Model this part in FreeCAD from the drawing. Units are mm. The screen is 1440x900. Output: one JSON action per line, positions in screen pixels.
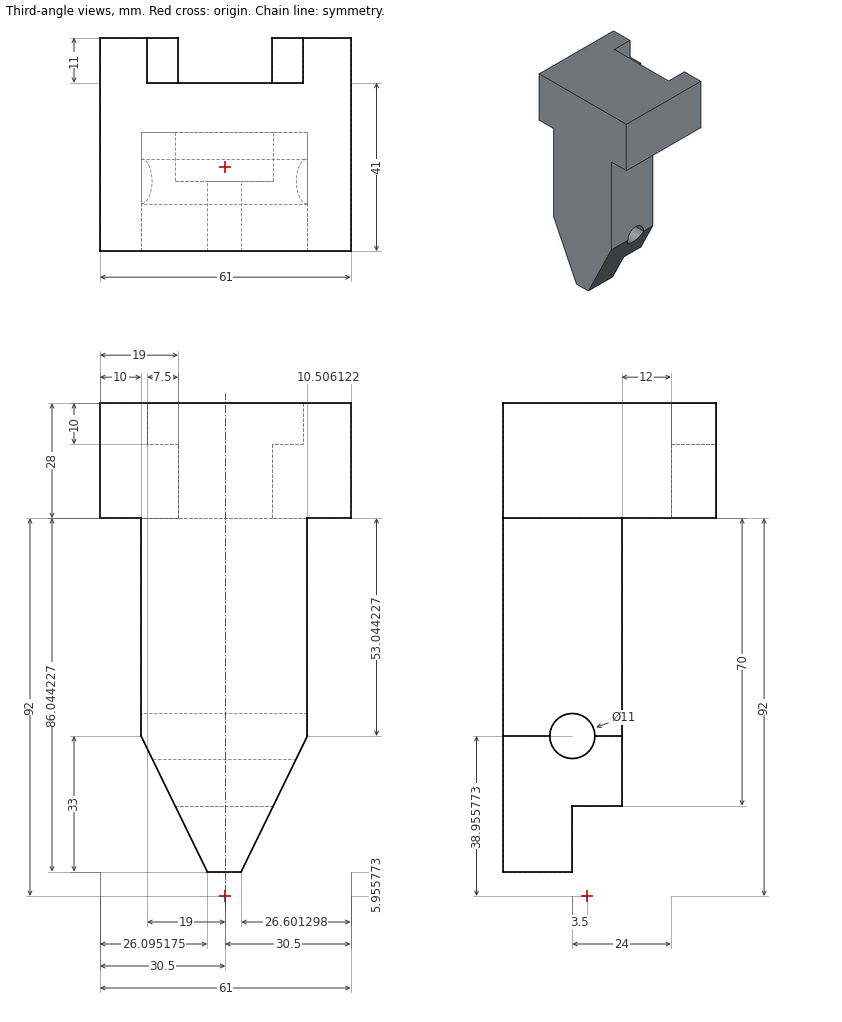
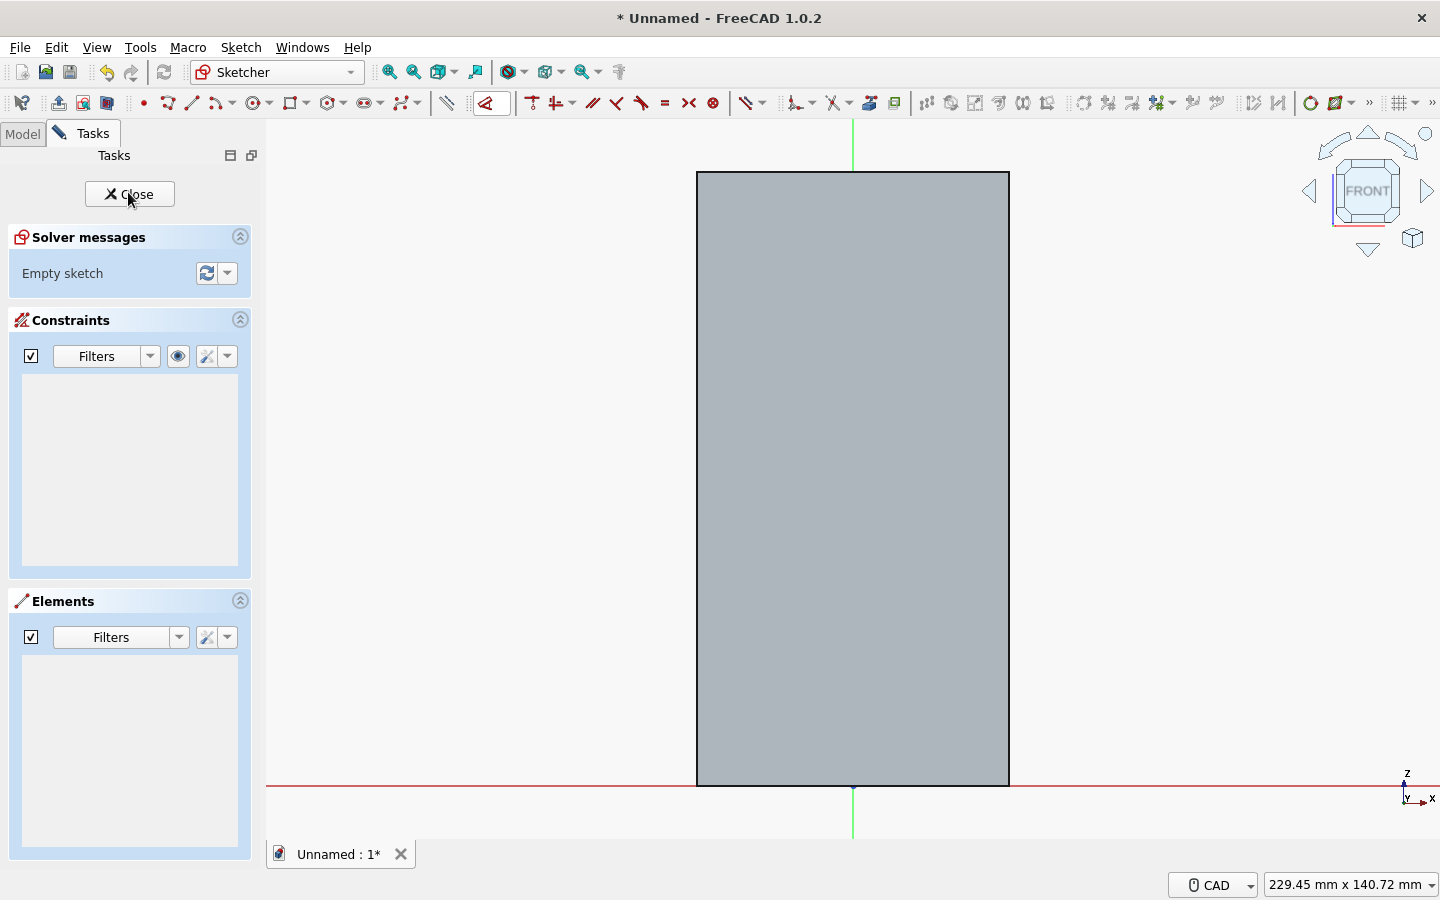
{"action": "left_click", "coordinate": [108, 104]}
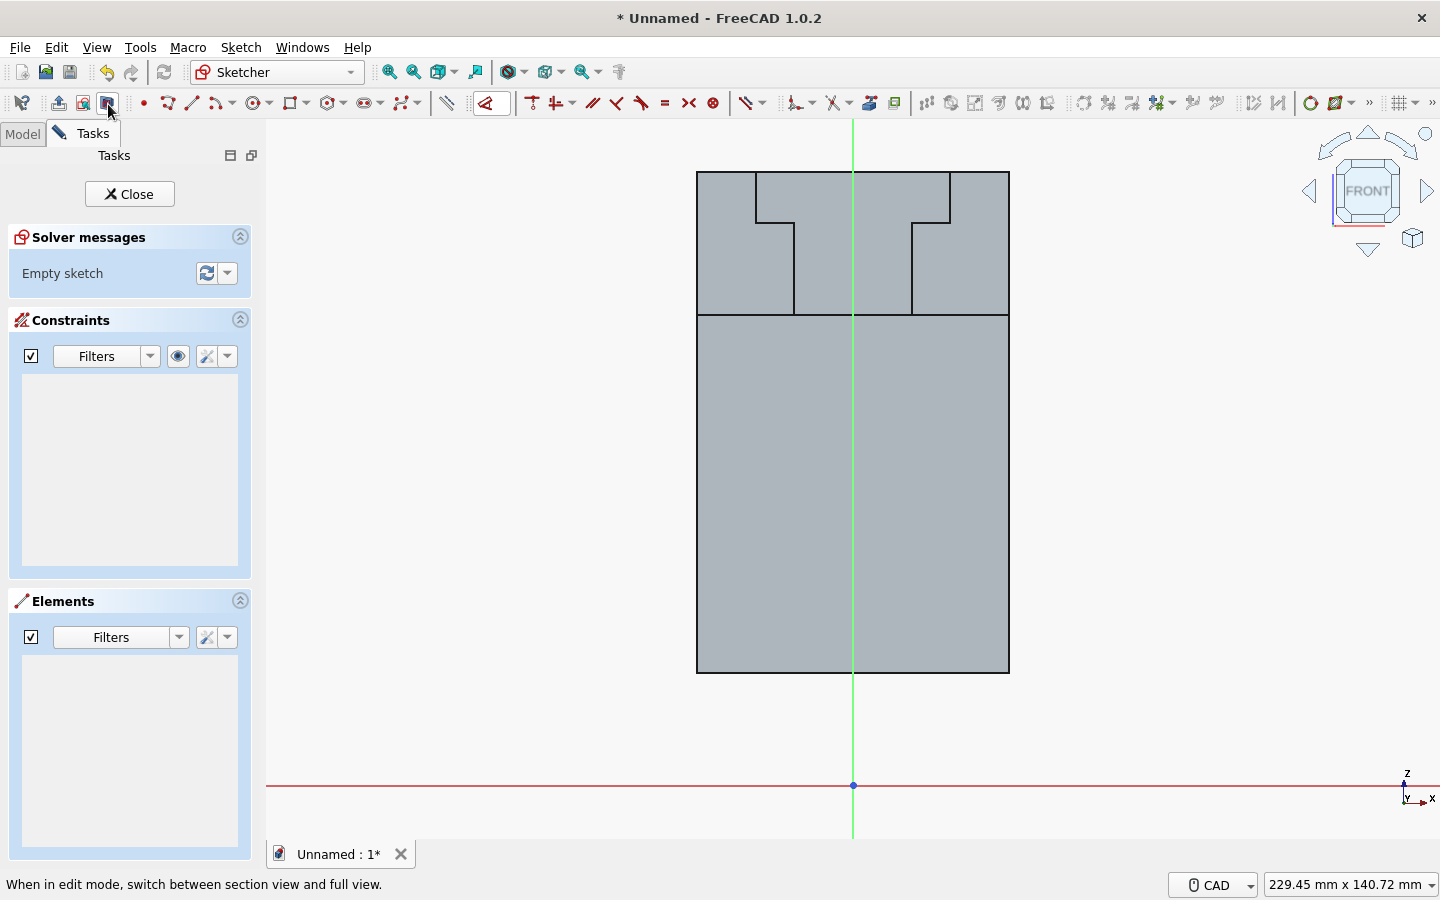
{"action": "left_click", "coordinate": [168, 104]}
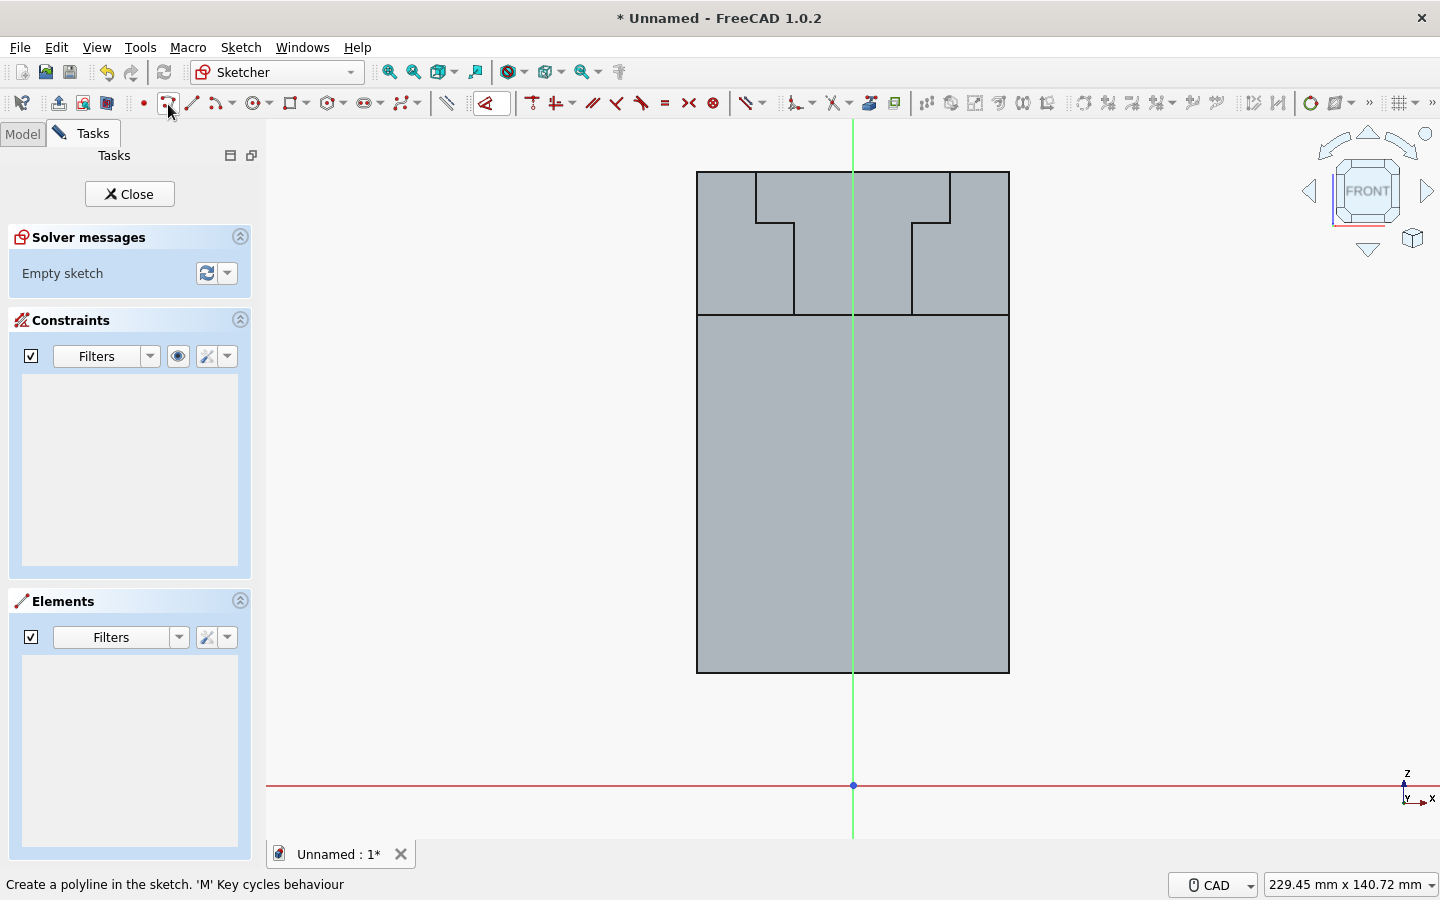
{"action": "left_click", "coordinate": [830, 756]}
{"action": "left_click", "coordinate": [697, 756]}
{"action": "left_click", "coordinate": [697, 315]}
{"action": "left_click", "coordinate": [748, 315]}
{"action": "left_click", "coordinate": [748, 587]}
{"action": "left_click", "coordinate": [830, 757]}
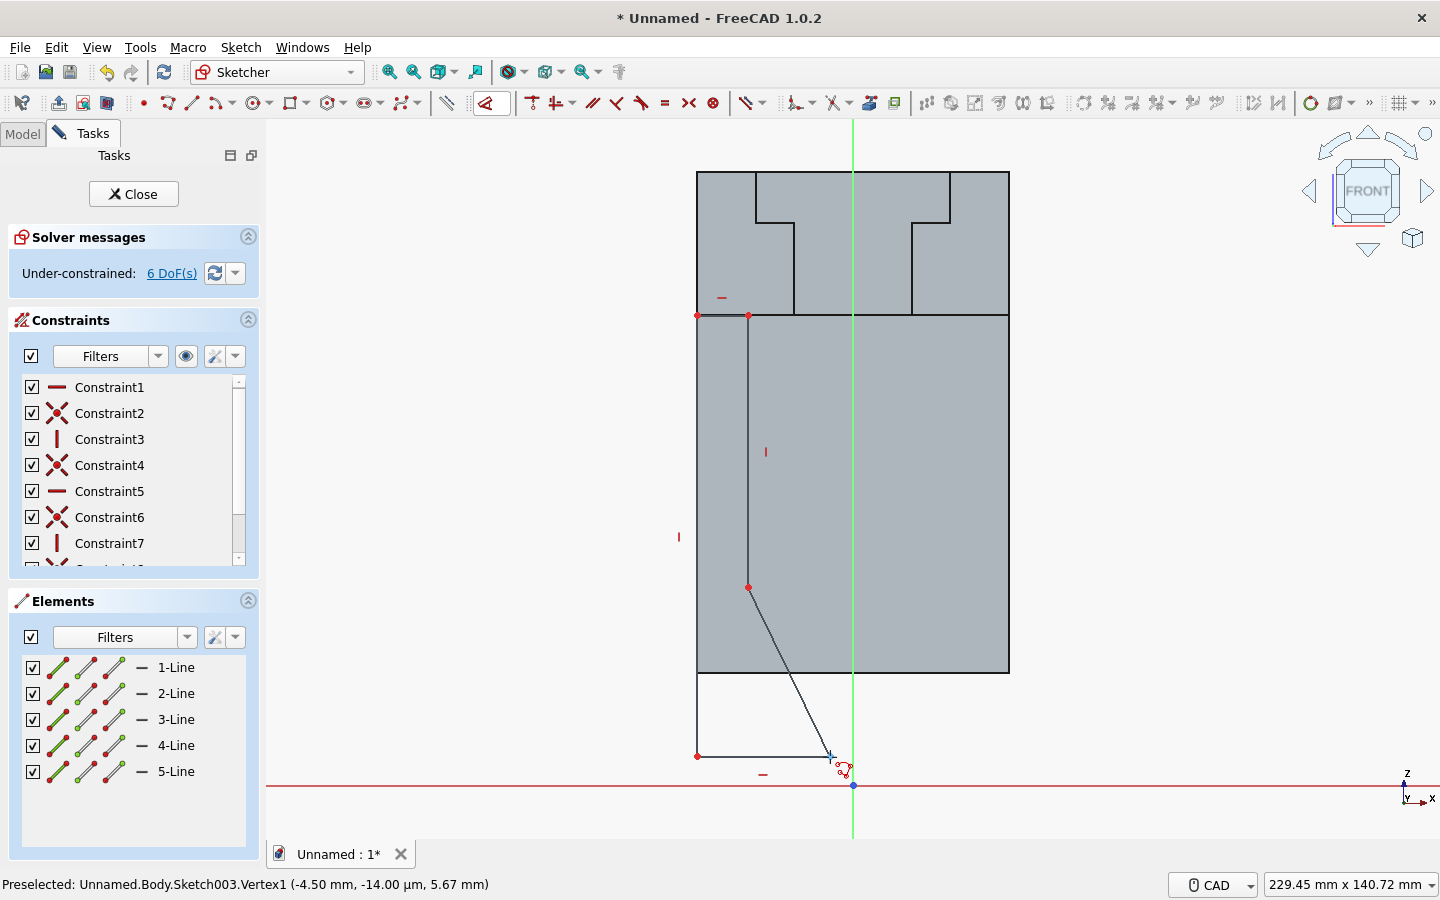
{"action": "left_click", "coordinate": [873, 756]}
{"action": "left_click", "coordinate": [955, 587]}
{"action": "left_click", "coordinate": [955, 315]}
{"action": "left_click", "coordinate": [1009, 315]}
{"action": "left_click", "coordinate": [1009, 756]}
{"action": "left_click", "coordinate": [873, 757]}
{"action": "key", "text": "Escape"}
{"action": "key", "text": "Escape"}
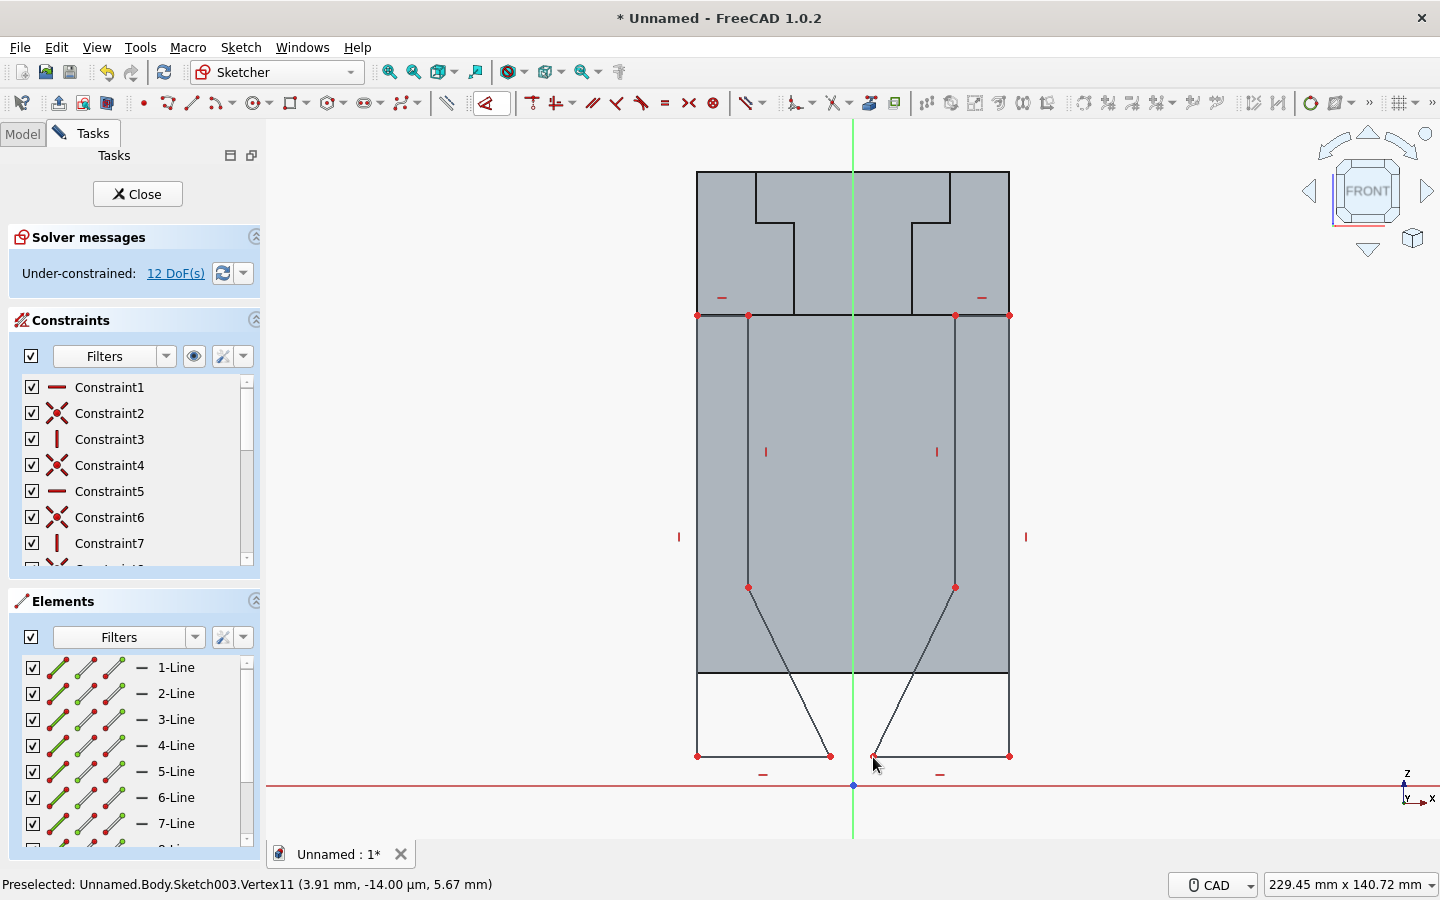
{"action": "left_click", "coordinate": [697, 316]}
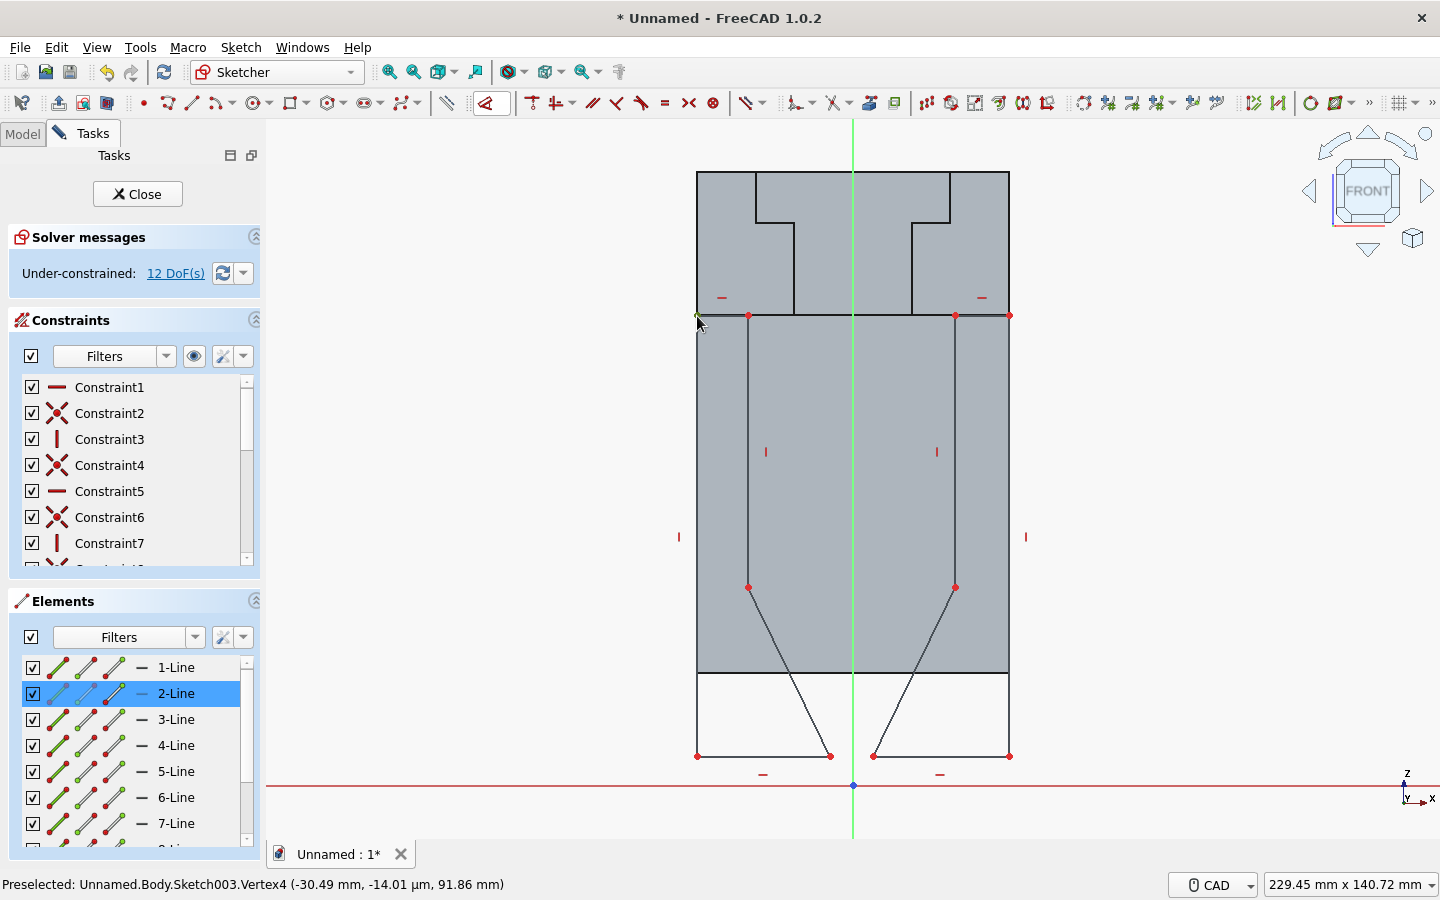
{"action": "left_click", "coordinate": [1009, 316]}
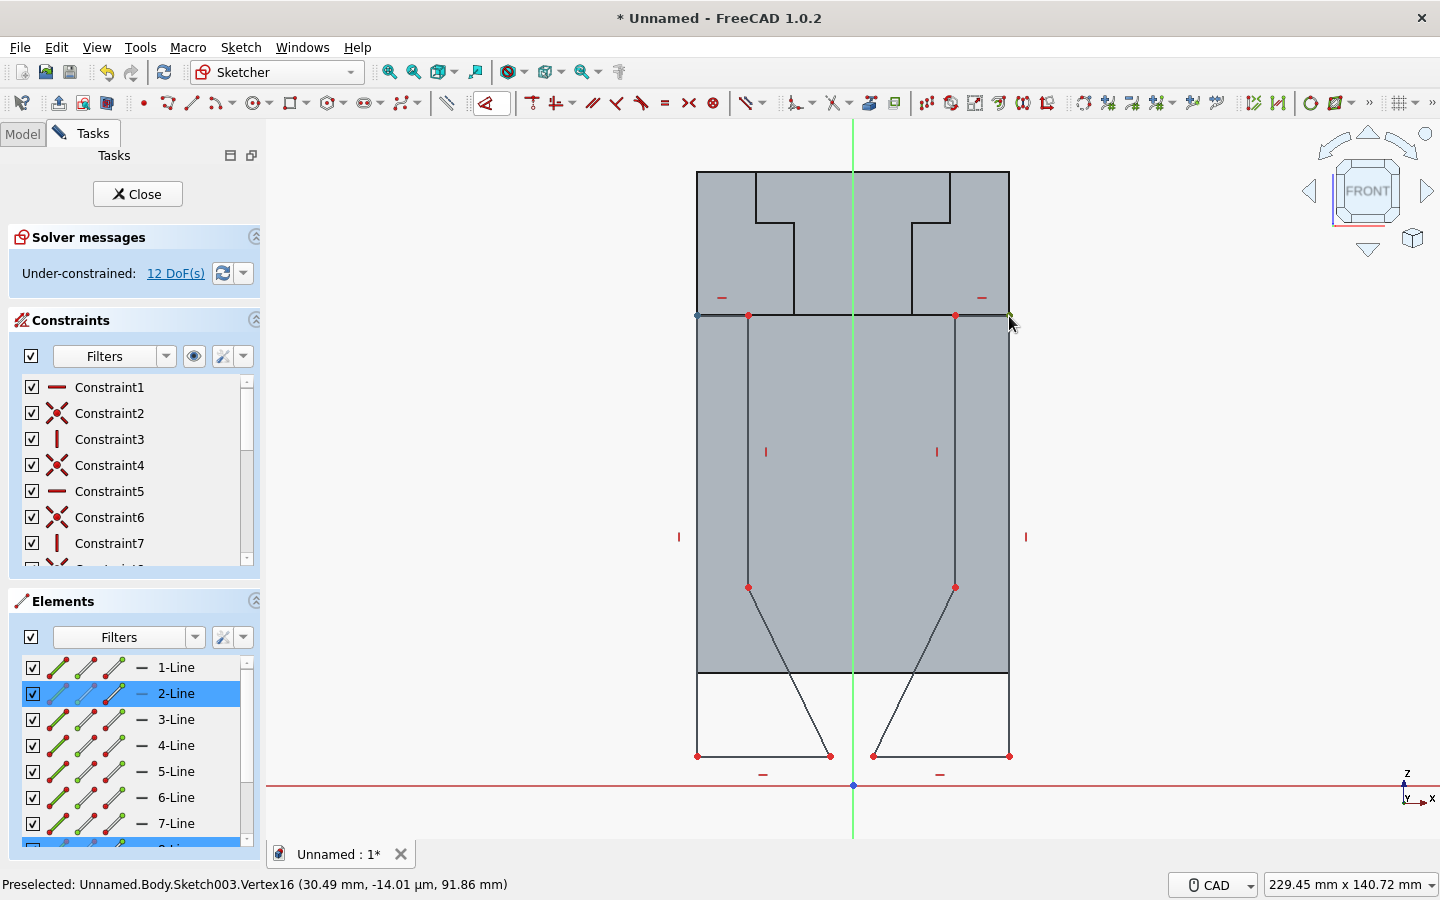
{"action": "left_click", "coordinate": [853, 716]}